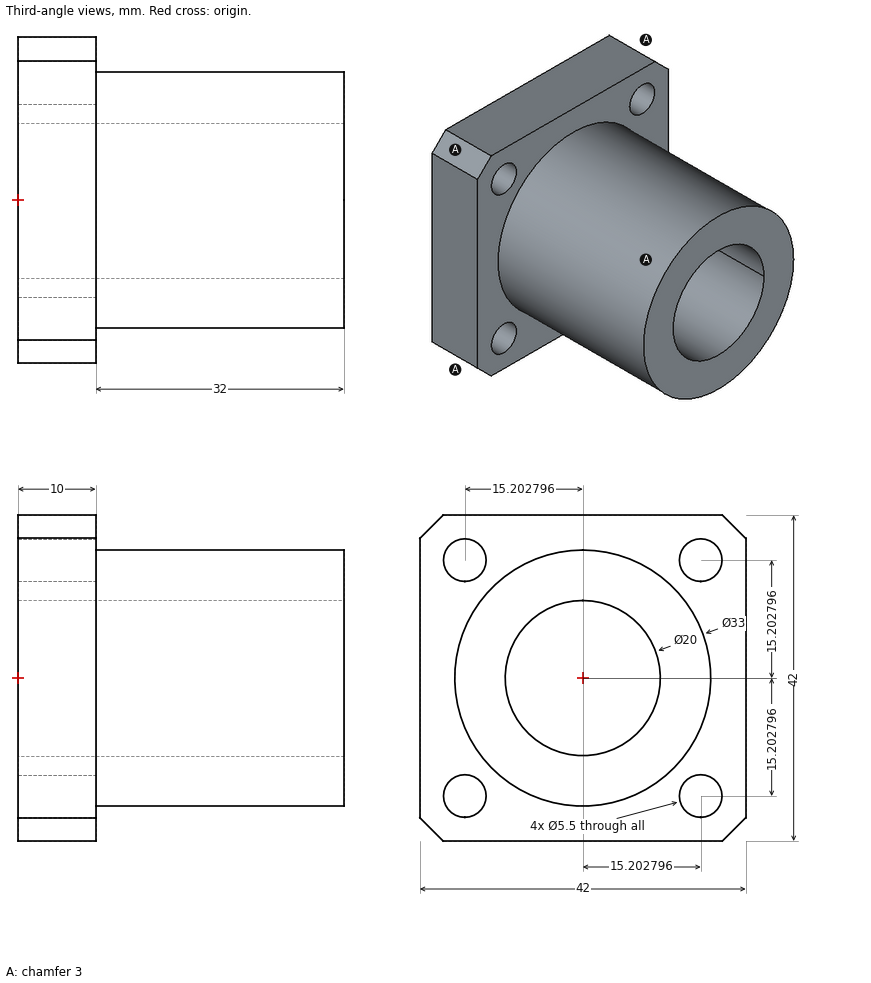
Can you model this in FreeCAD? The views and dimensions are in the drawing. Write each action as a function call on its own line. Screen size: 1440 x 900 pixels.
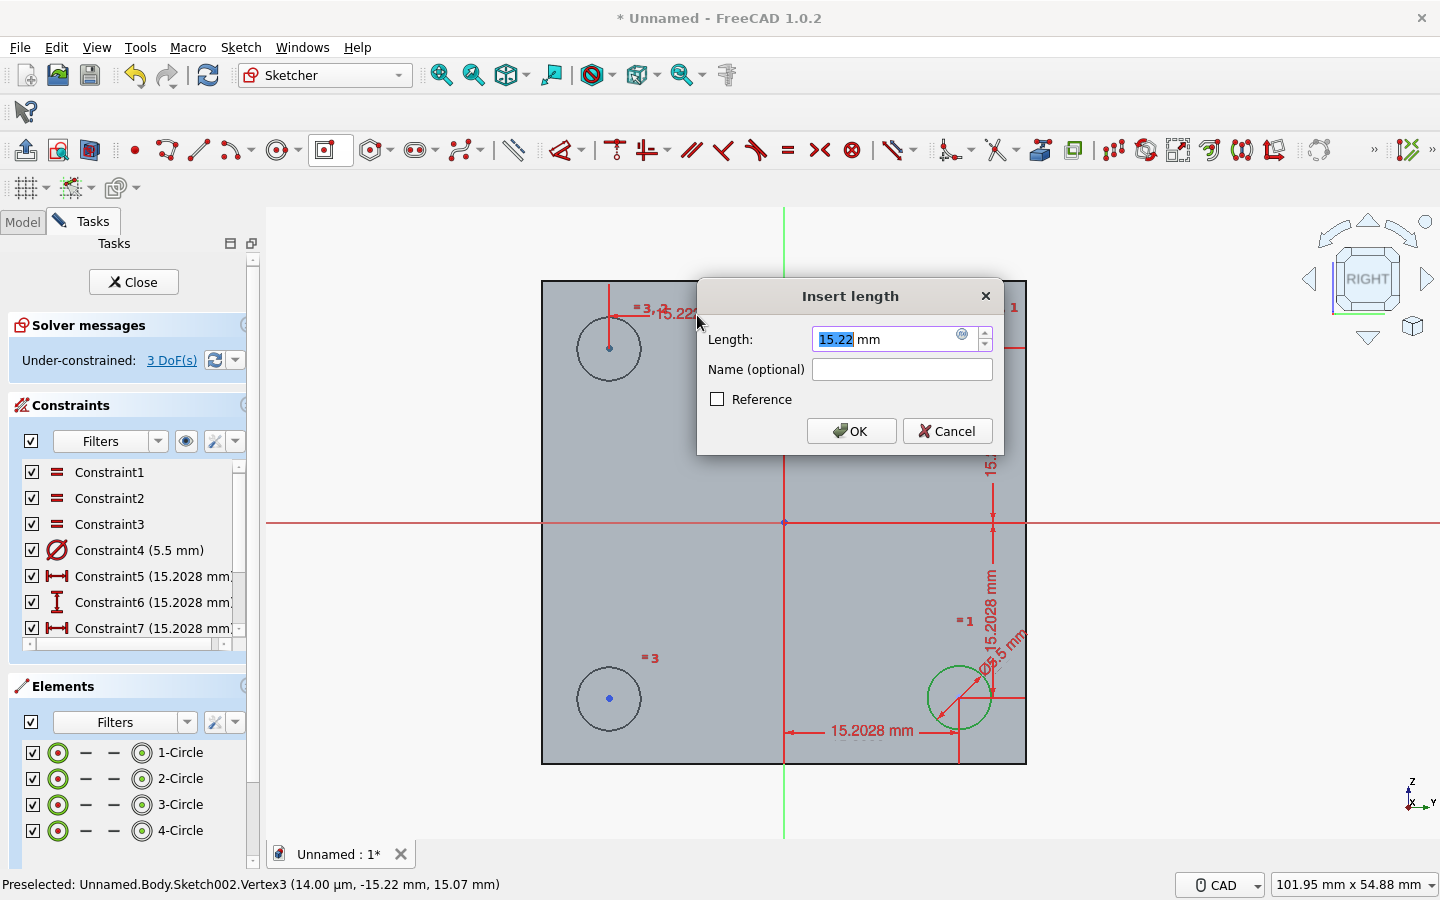
text(15.202796)
key(Return)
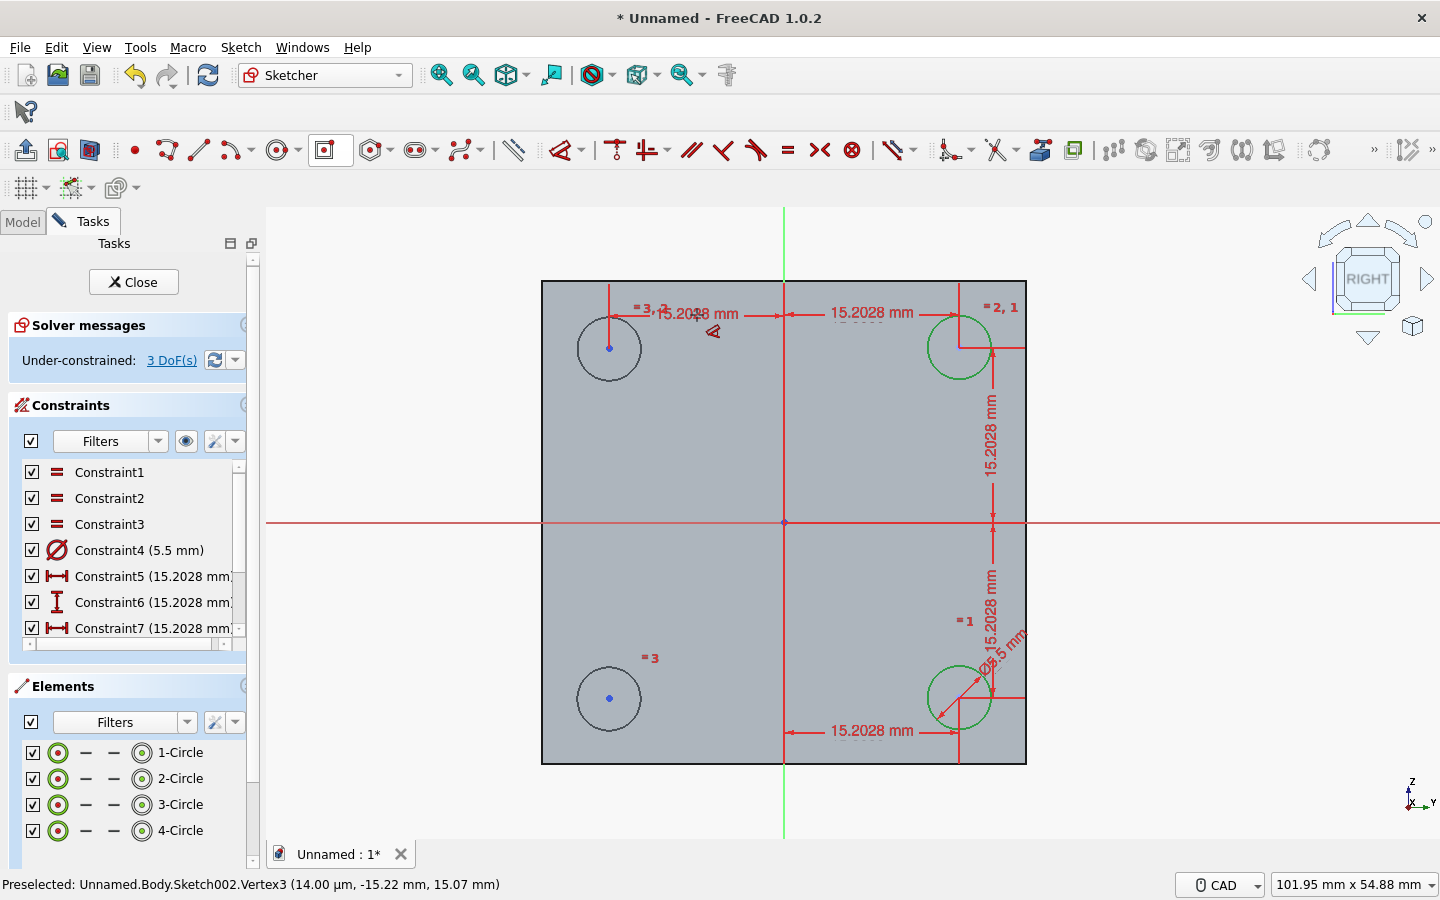
click(609, 349)
click(575, 436)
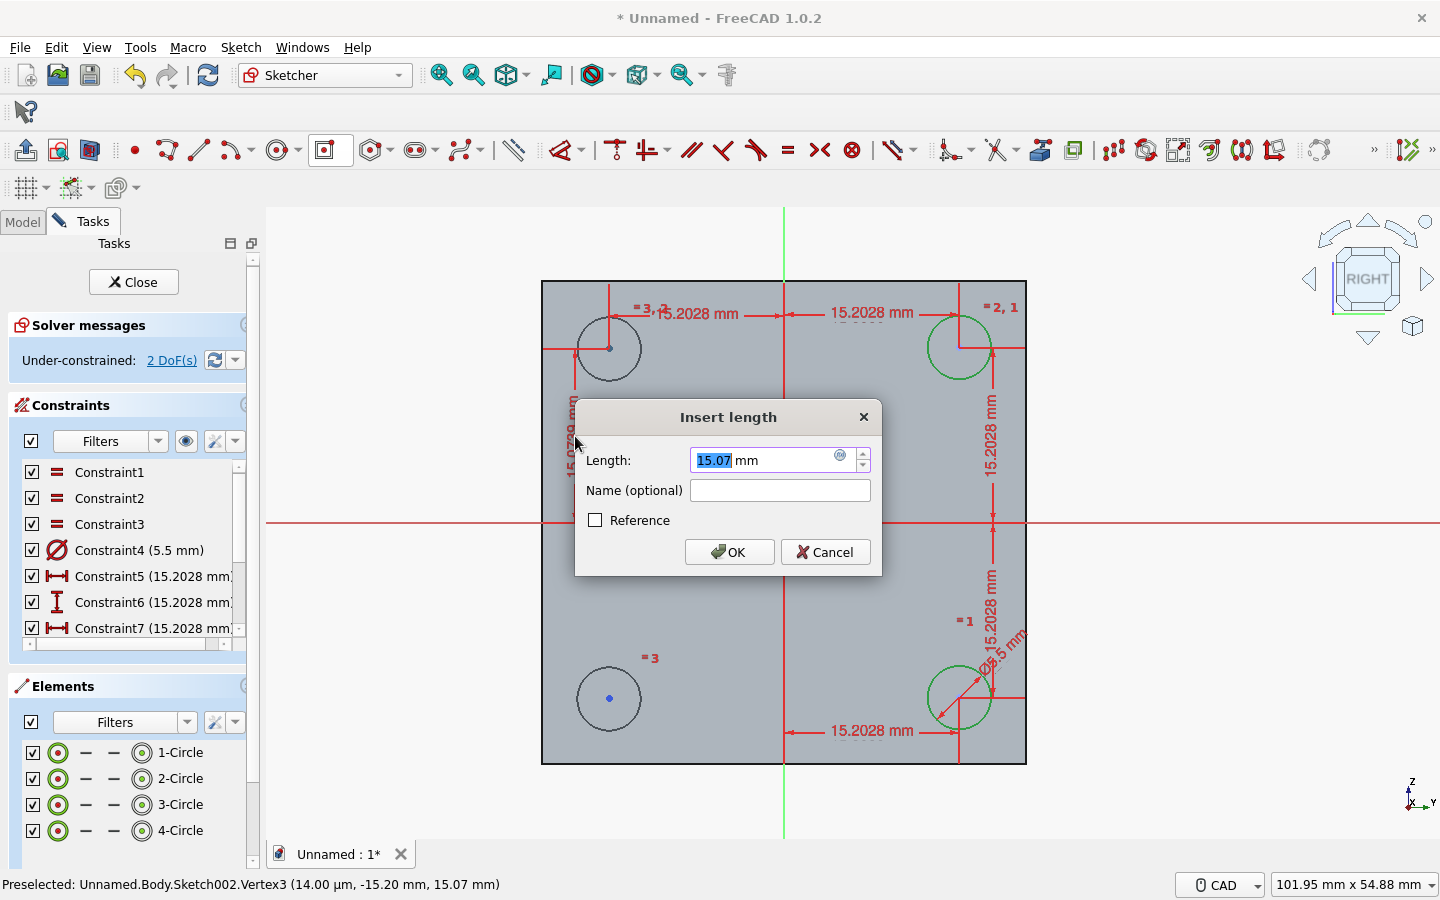
text(15.202796)
key(Return)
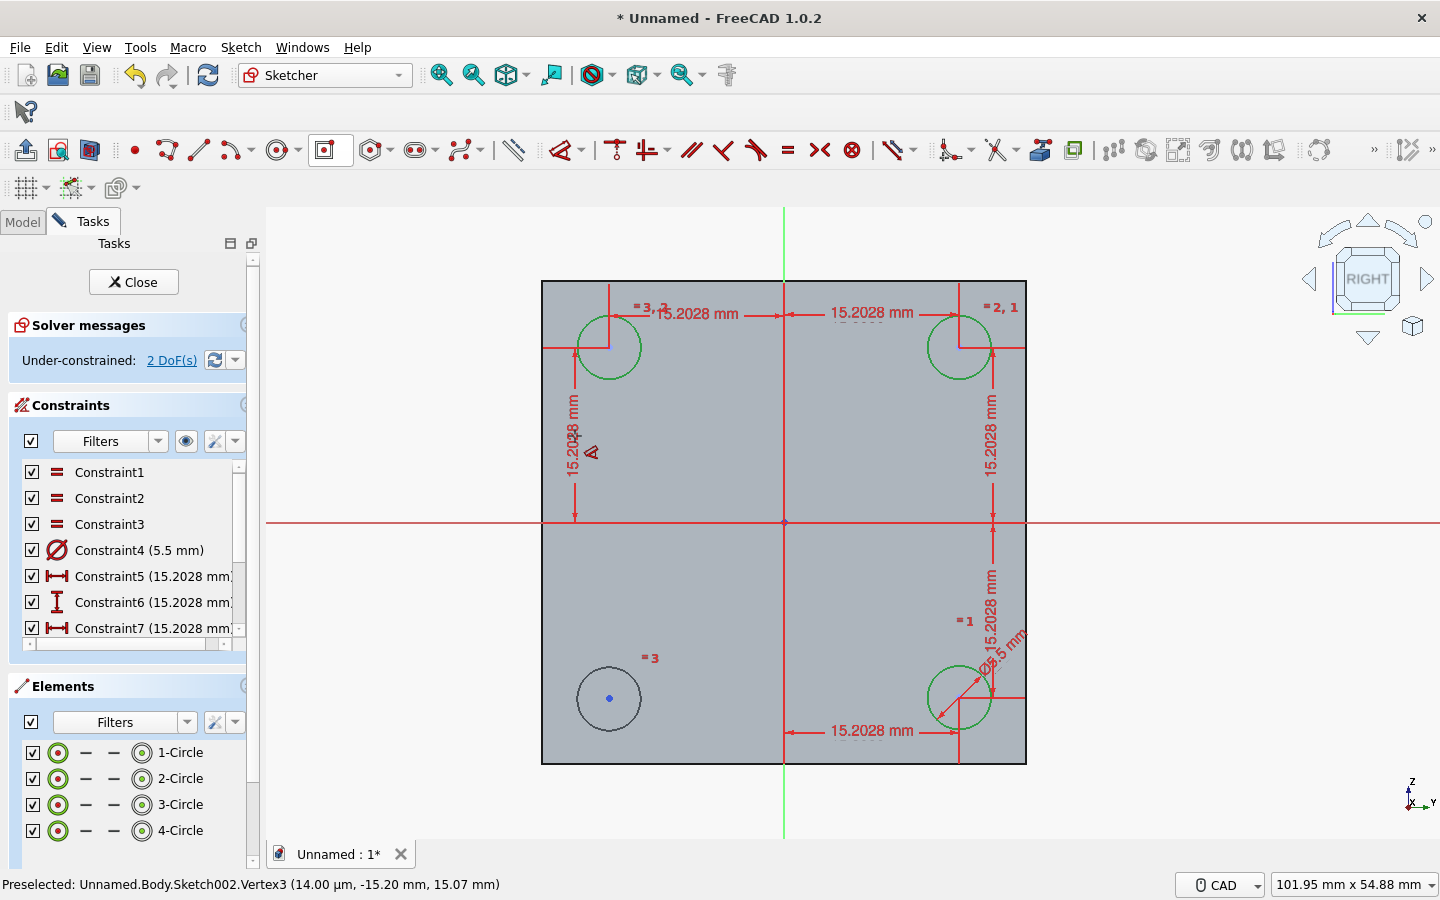
click(609, 699)
click(697, 733)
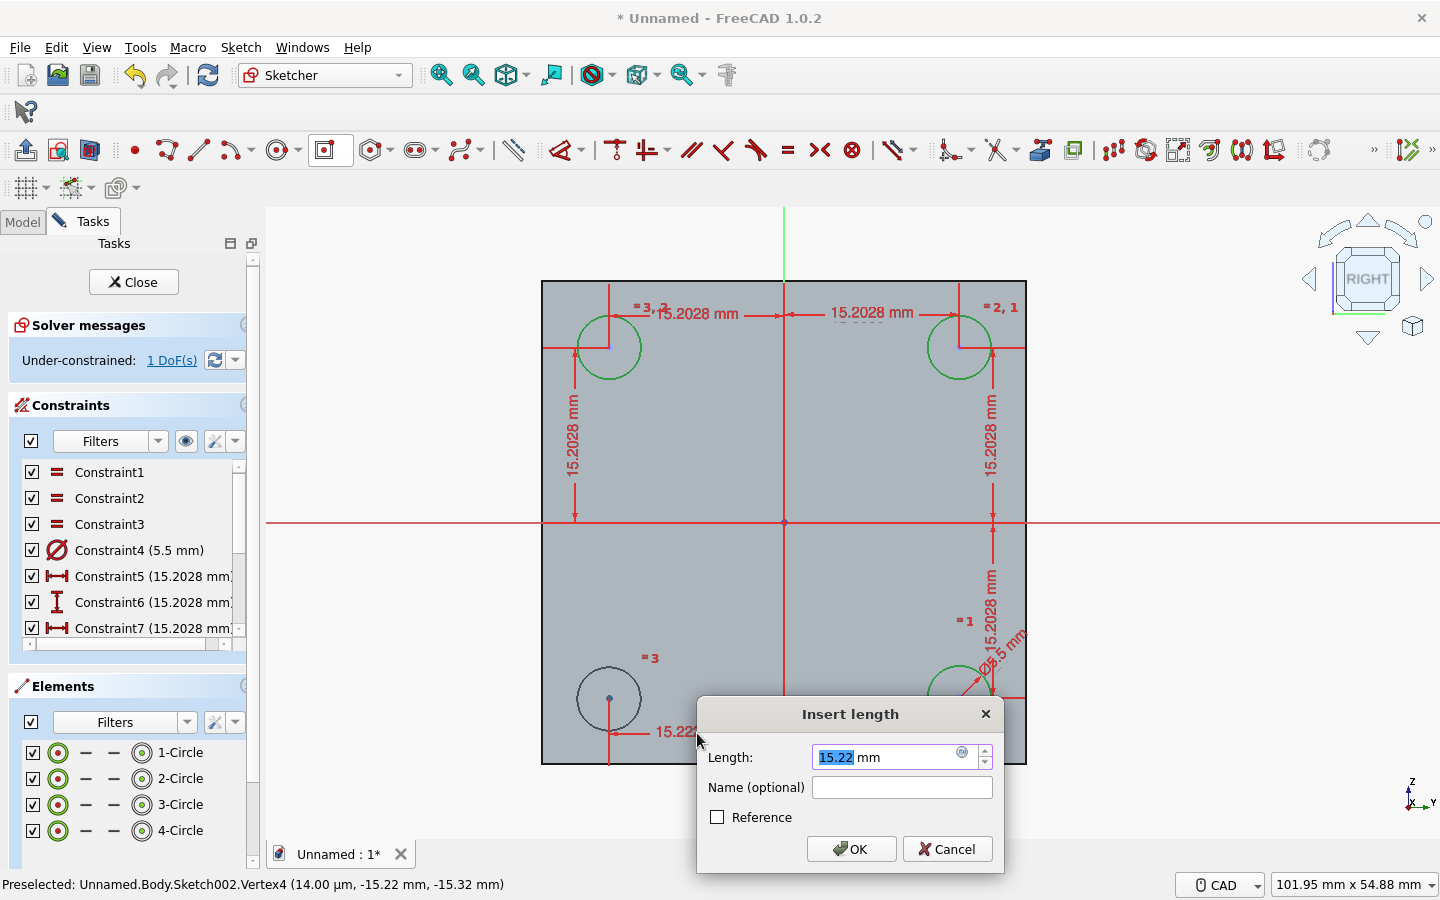
text(15.202796)
key(Return)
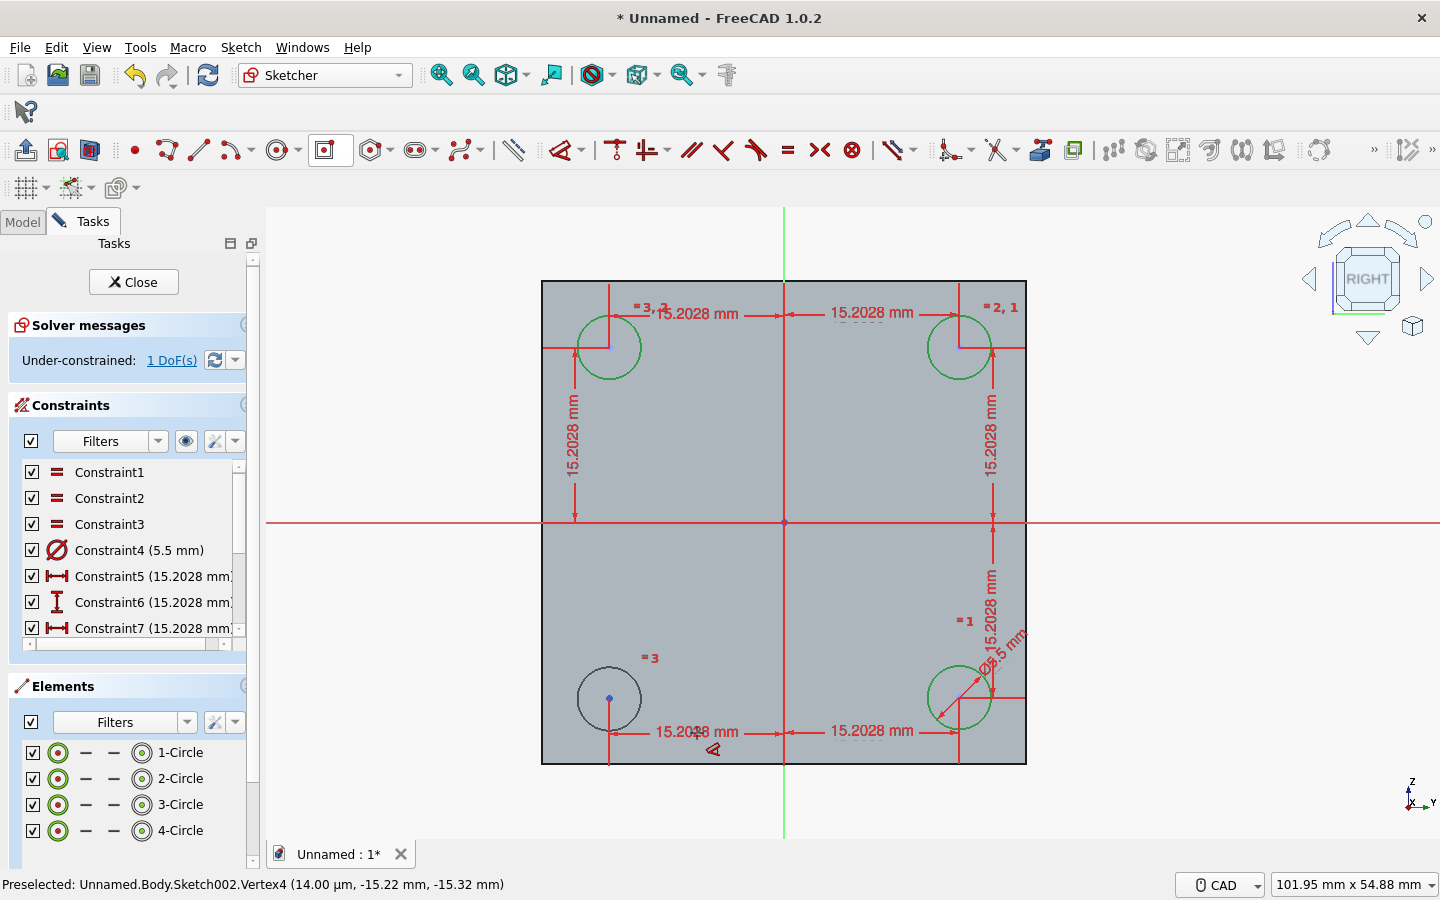
click(609, 699)
click(575, 611)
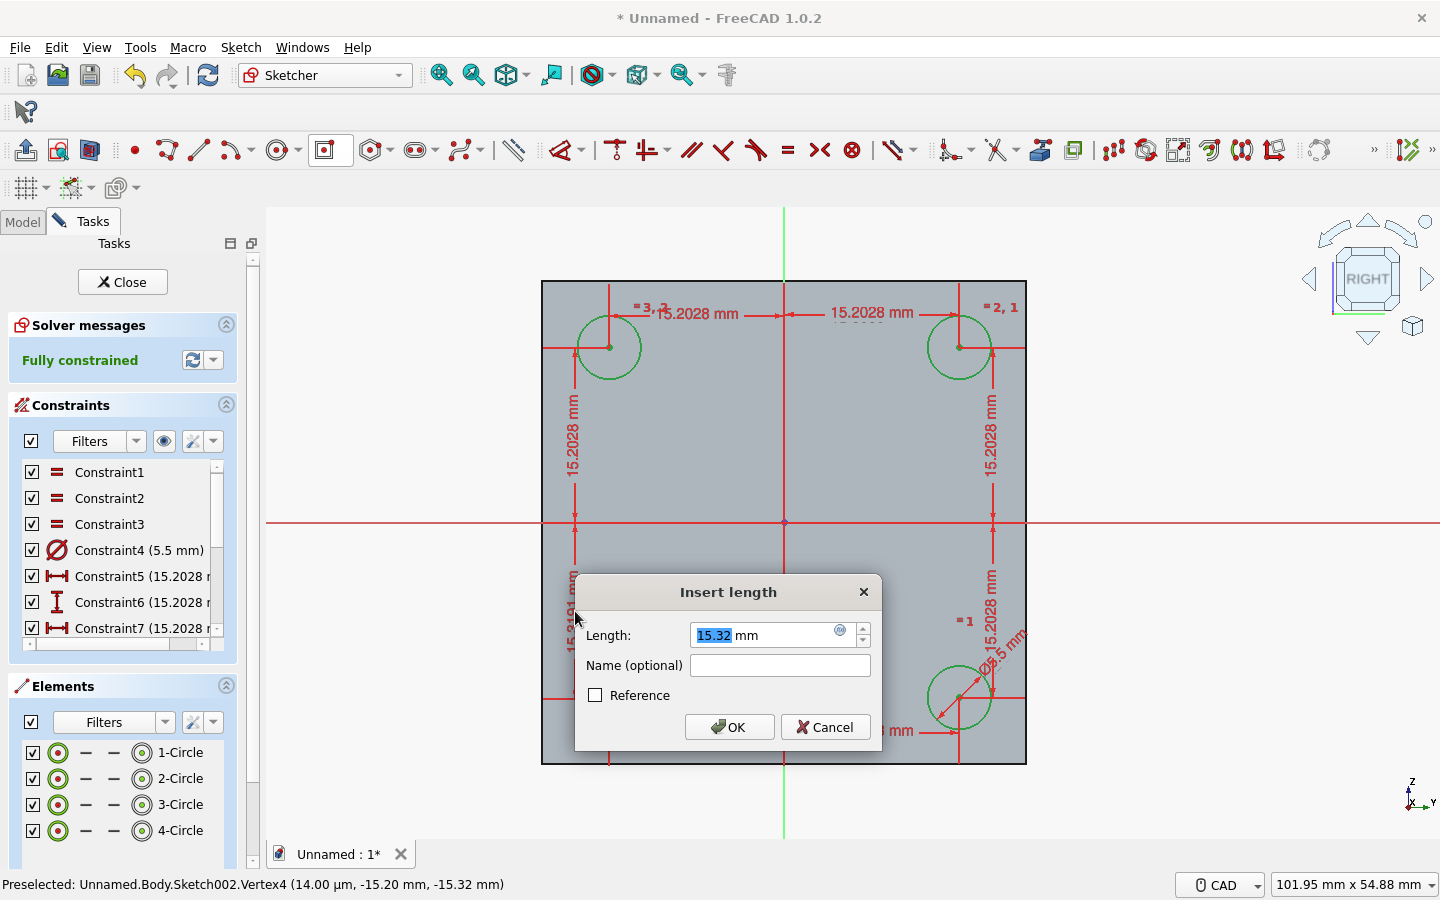
text(15.202796)
key(Return)
key(Escape)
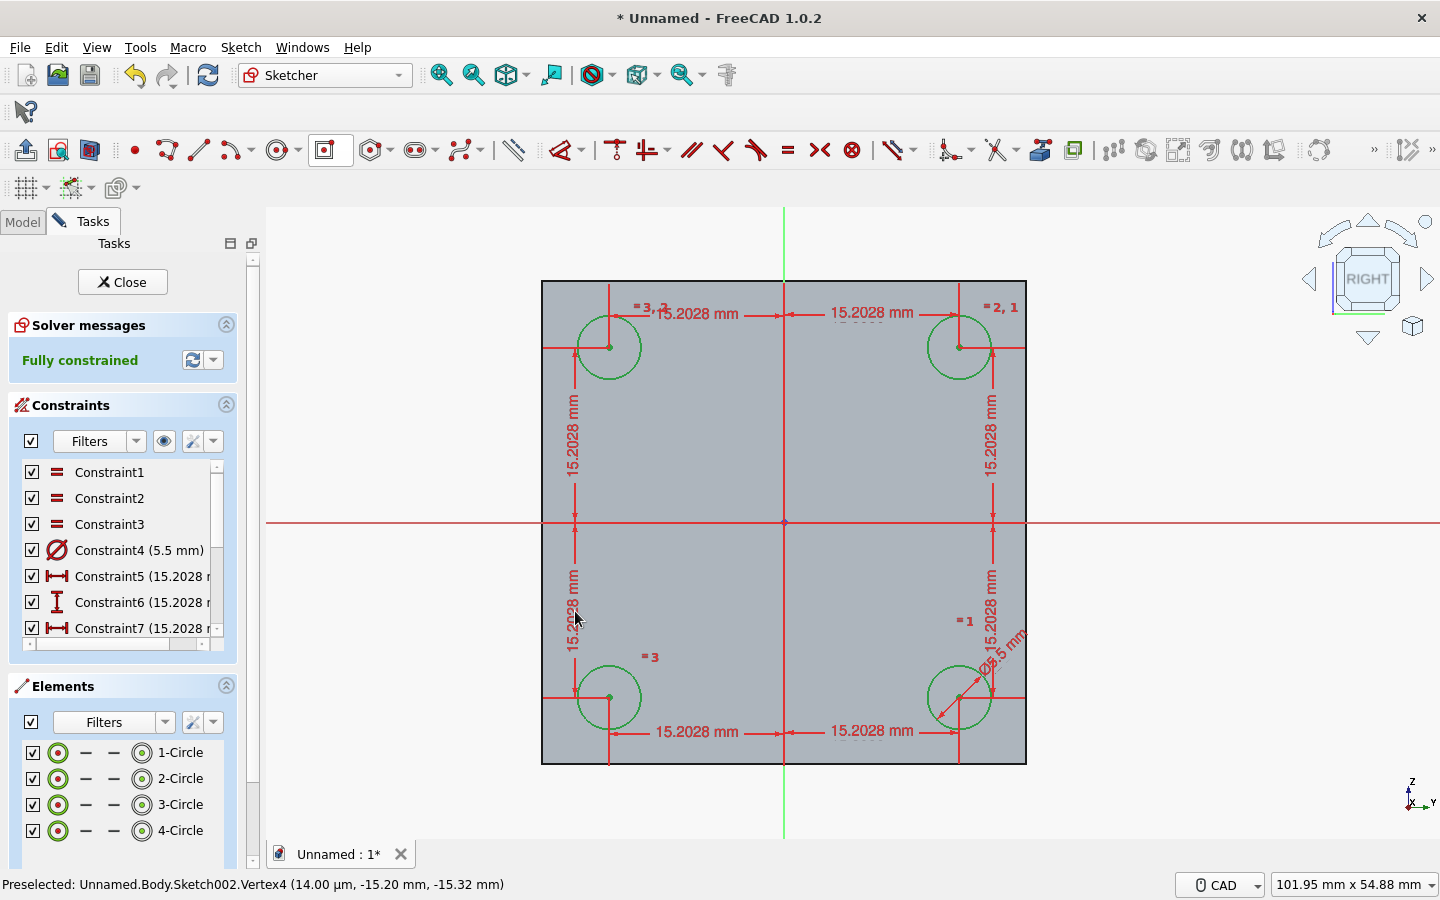
click(123, 282)